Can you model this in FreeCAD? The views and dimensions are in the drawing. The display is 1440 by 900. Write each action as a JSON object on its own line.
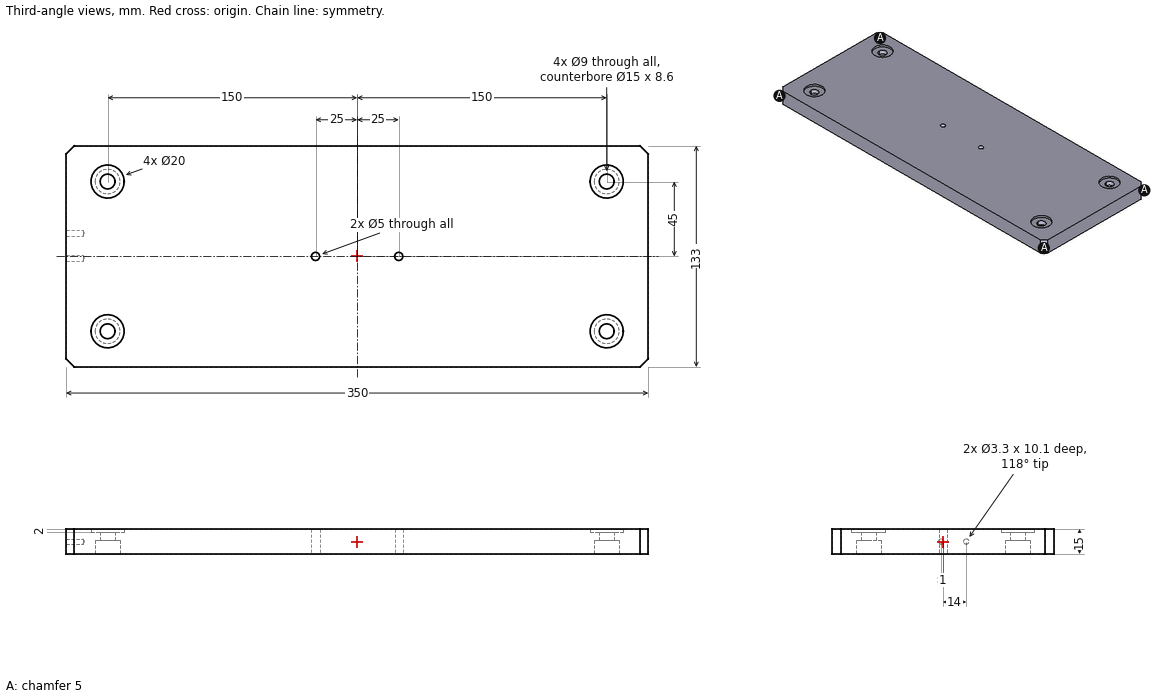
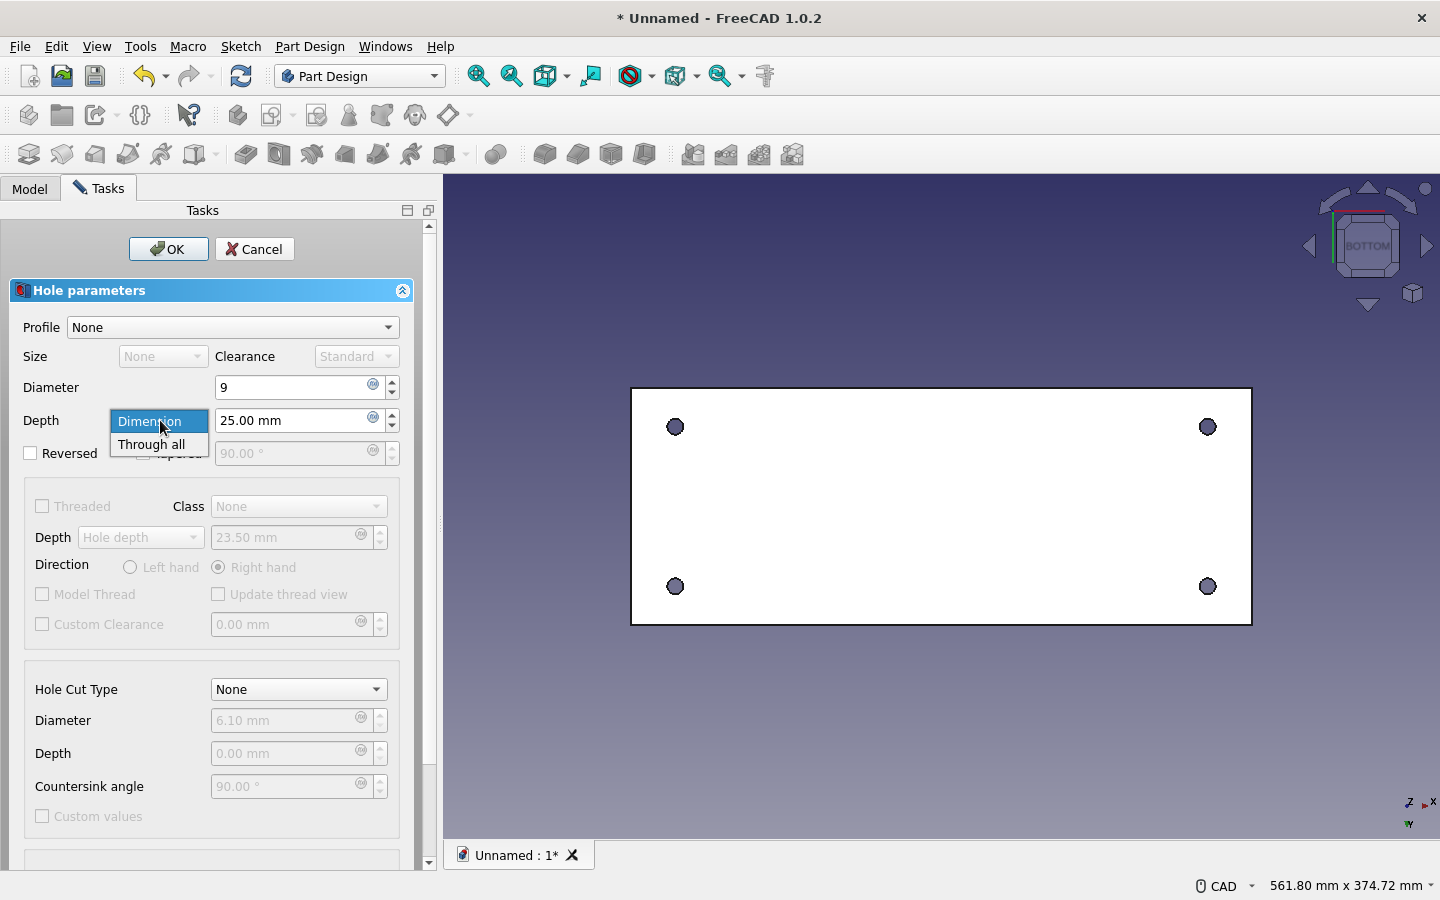
{"action": "left_click", "coordinate": [158, 444]}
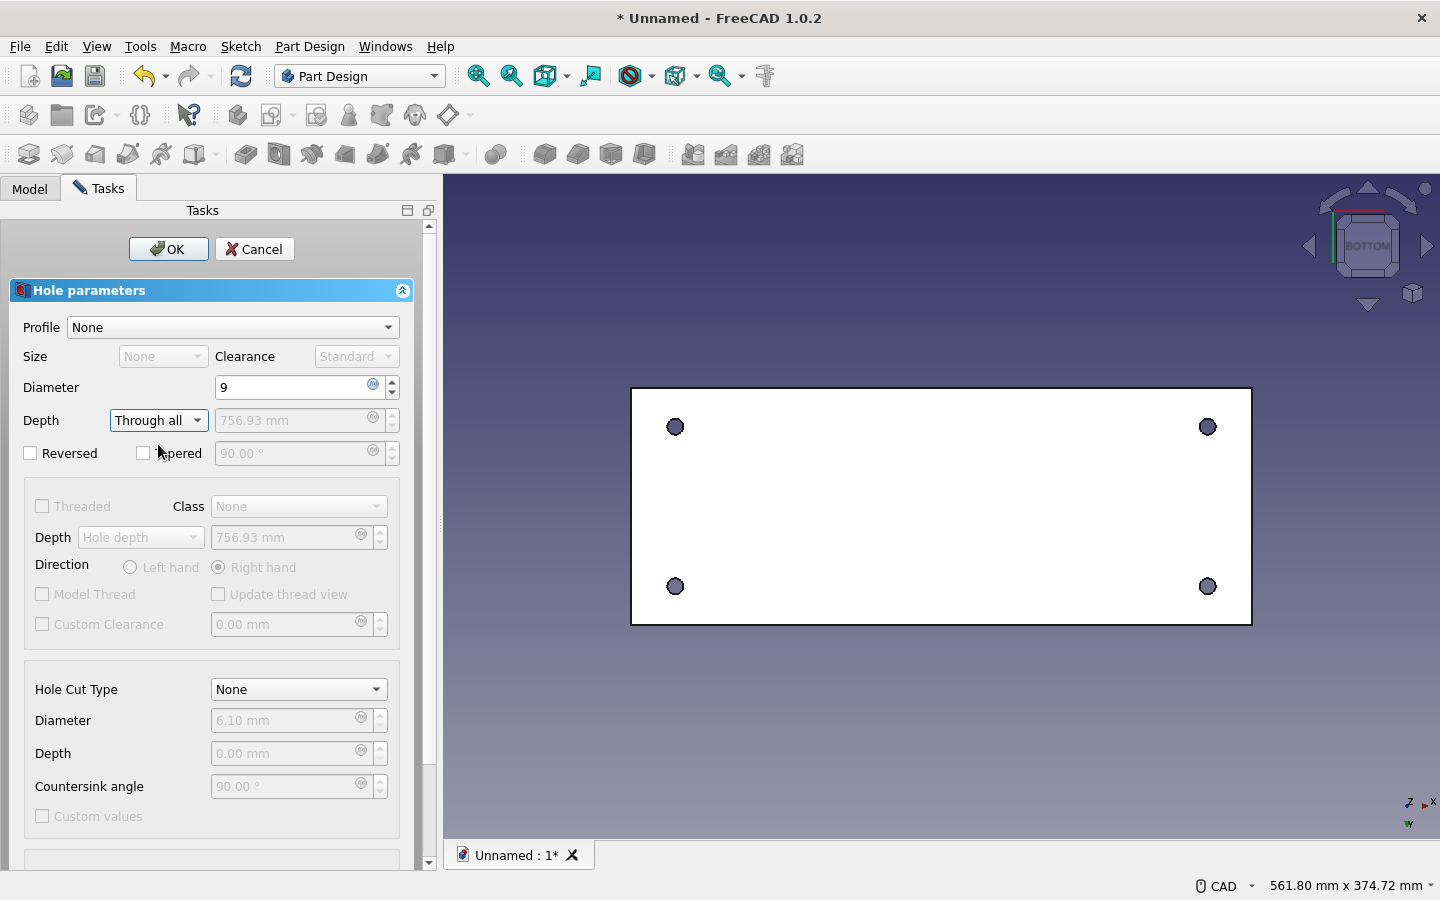
{"action": "left_click", "coordinate": [300, 690]}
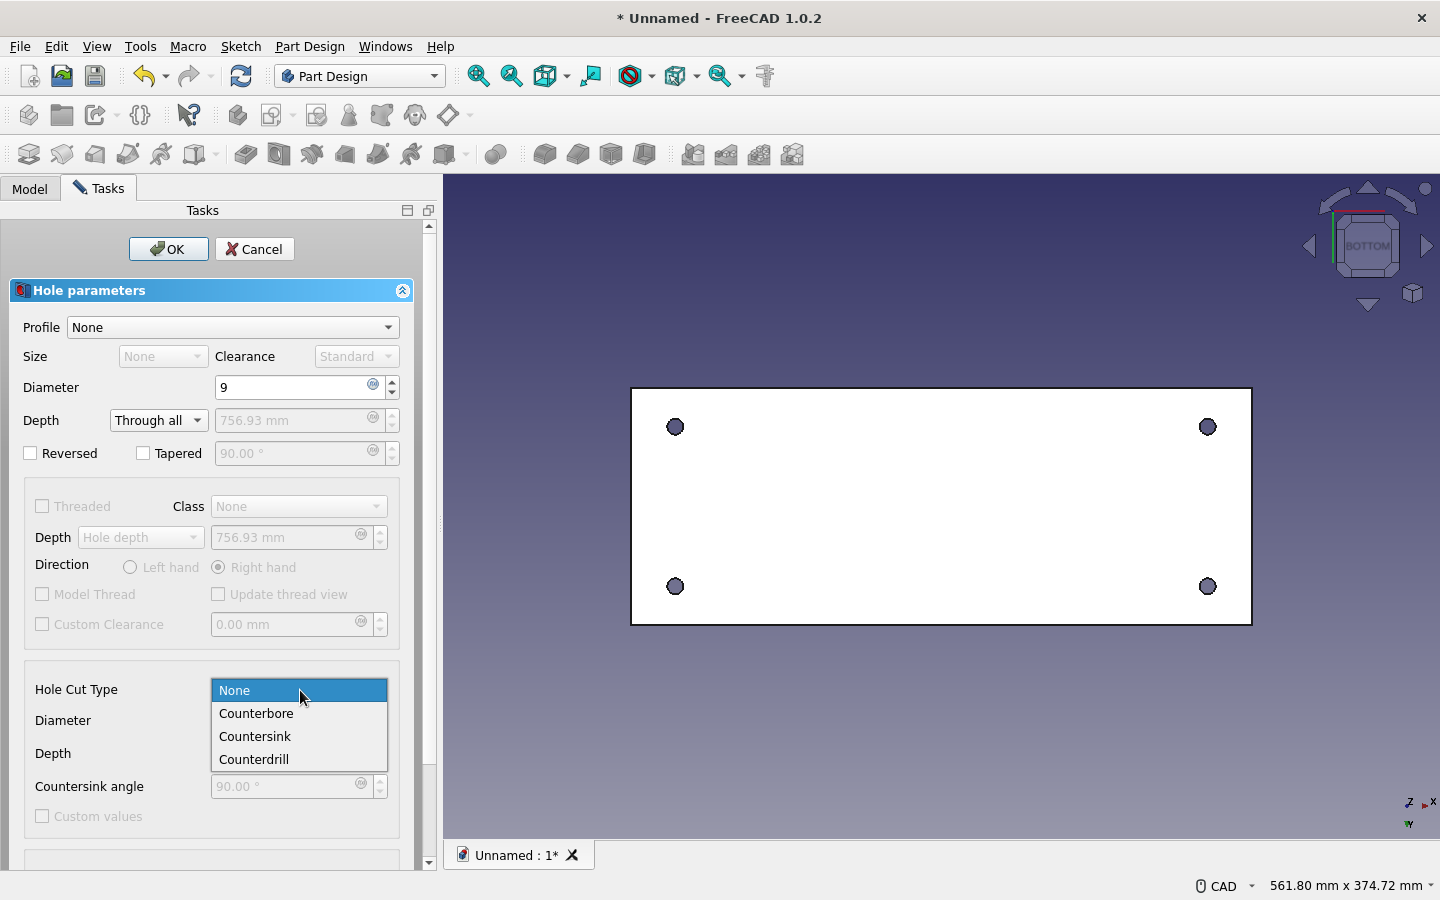
{"action": "left_click", "coordinate": [298, 714]}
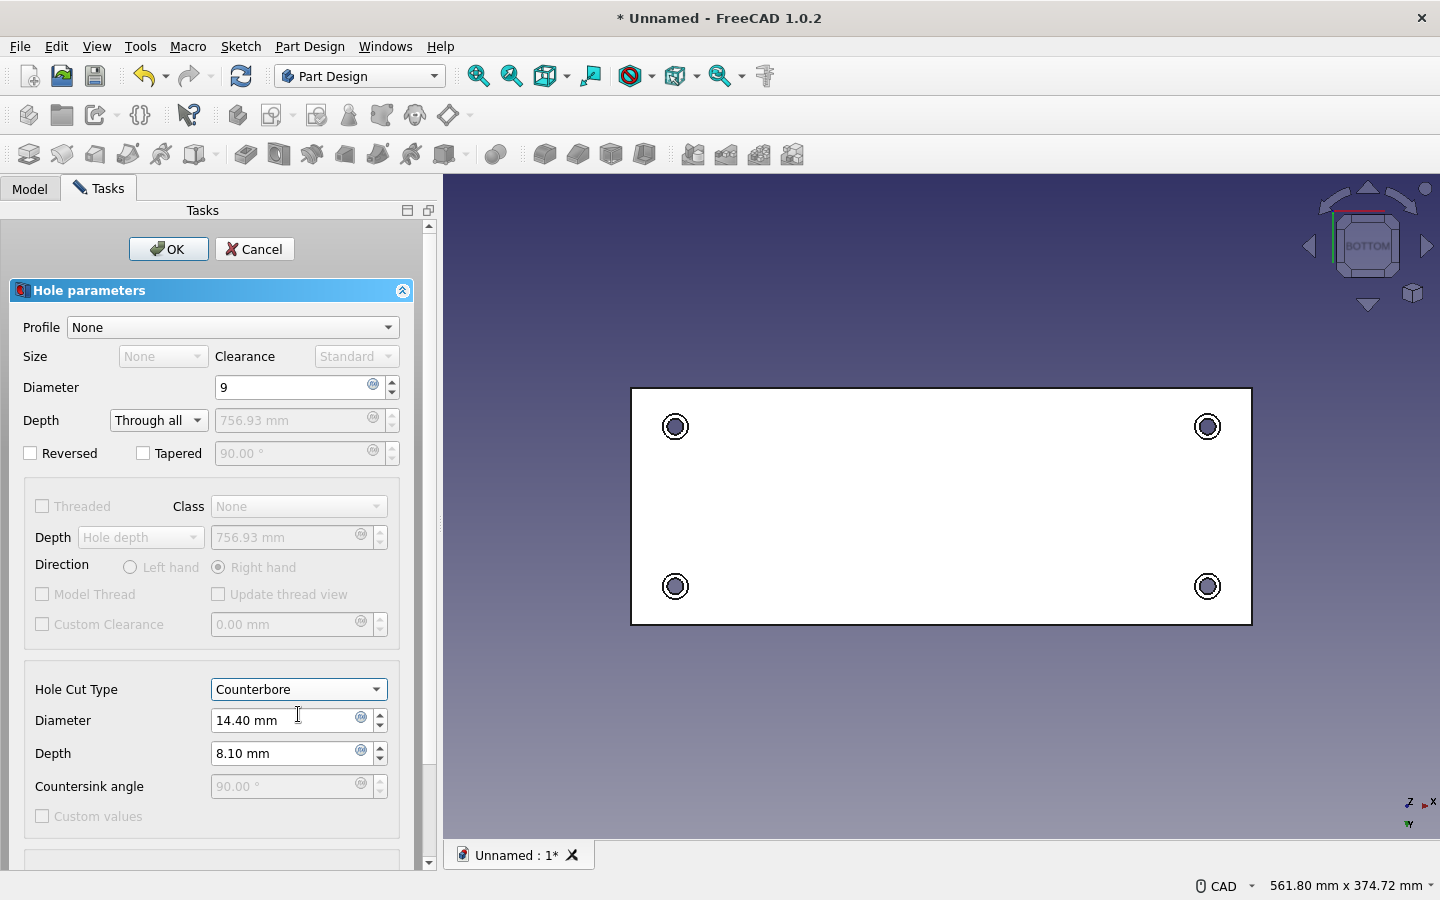
{"action": "triple_click", "coordinate": [292, 720]}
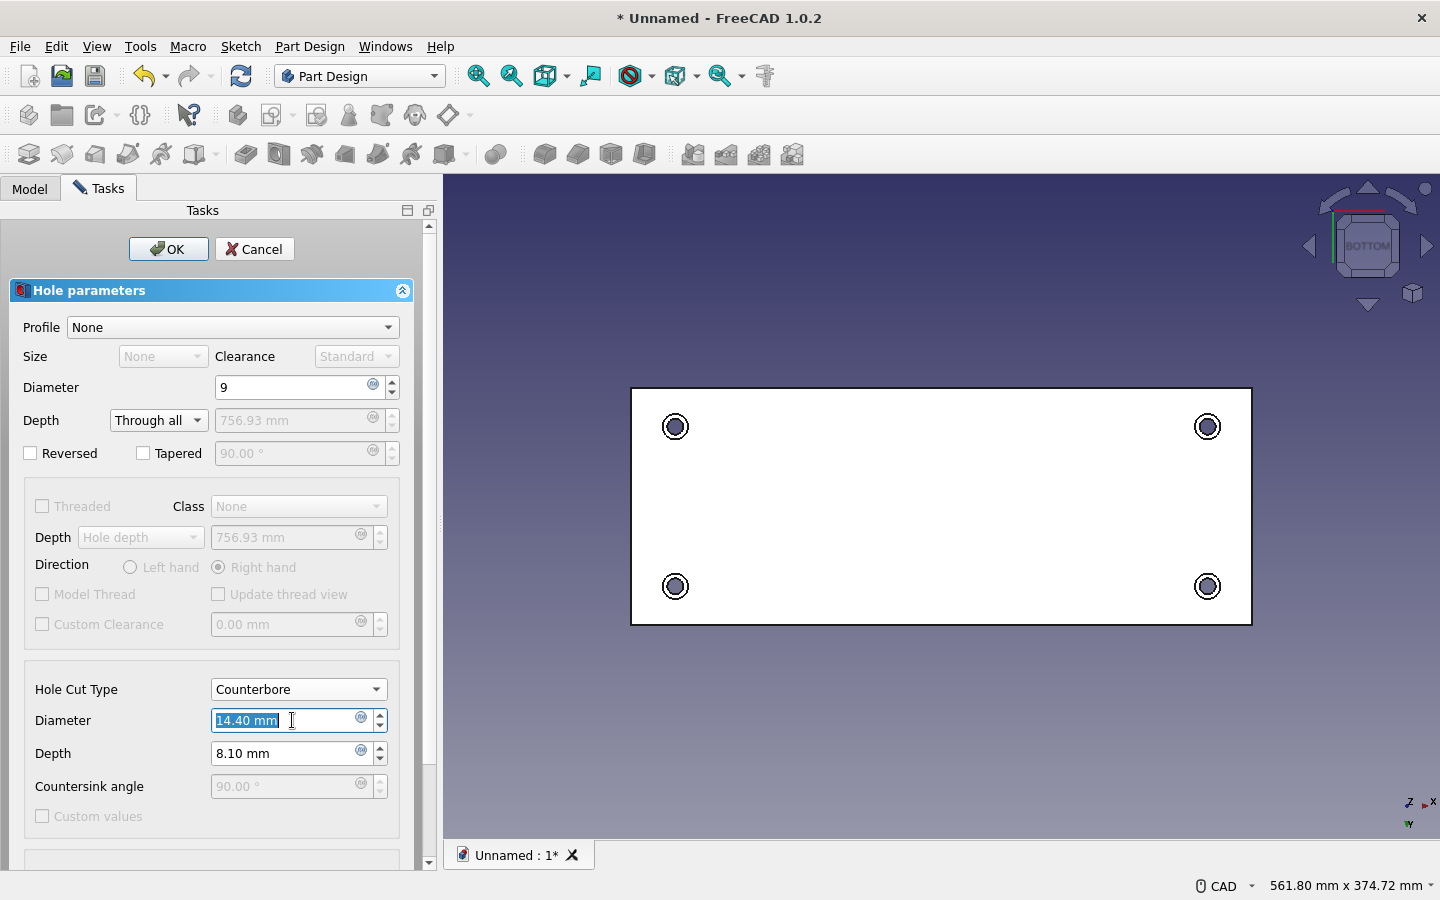
{"action": "type", "text": "15"}
{"action": "key", "text": "Tab"}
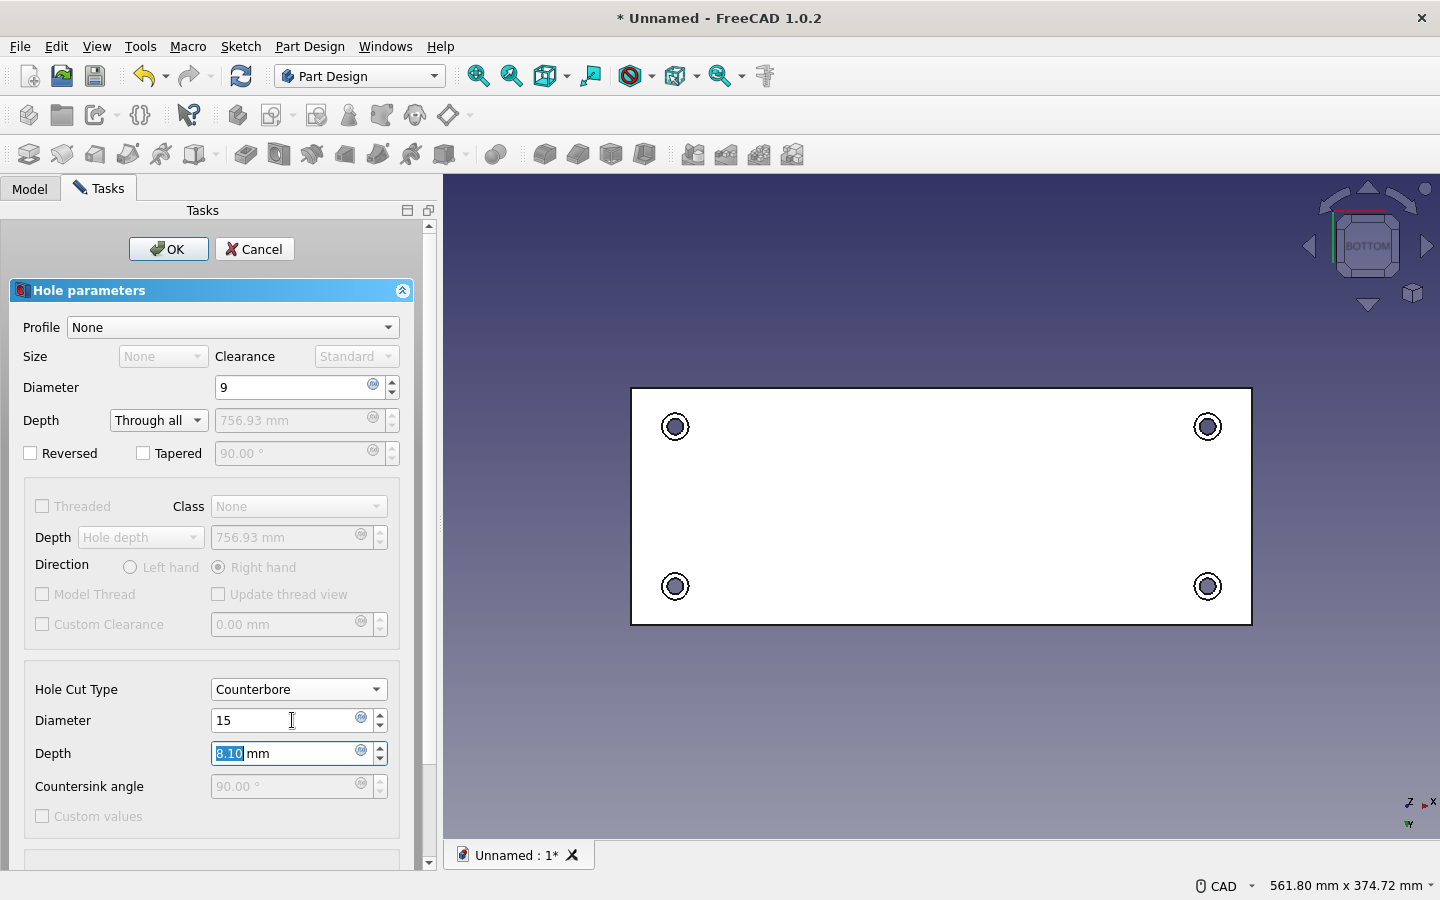
{"action": "type", "text": "8.6"}
{"action": "key", "text": "Tab"}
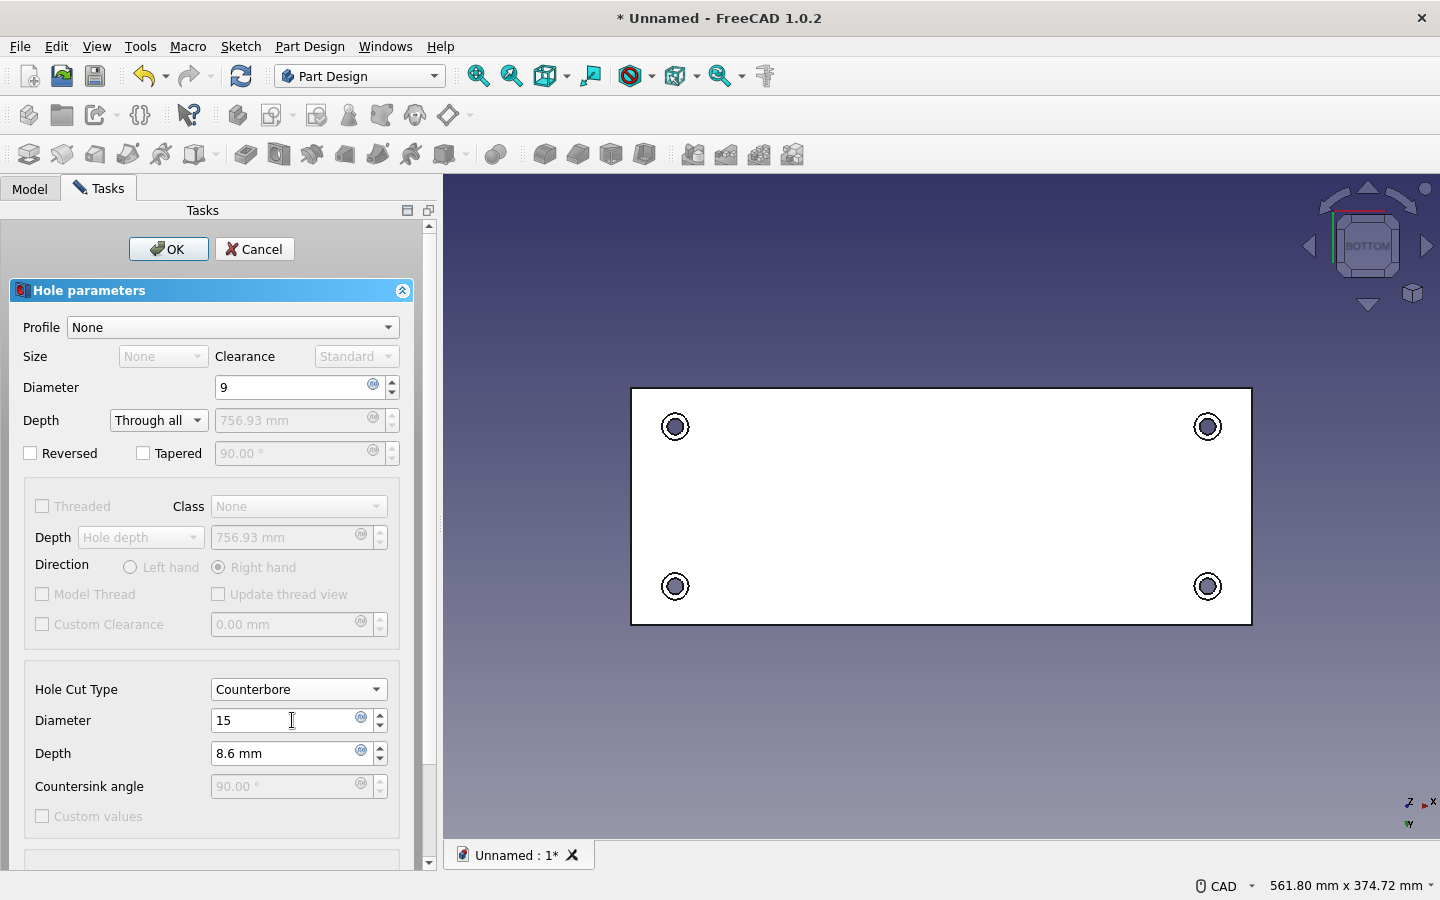
{"action": "left_click", "coordinate": [169, 249]}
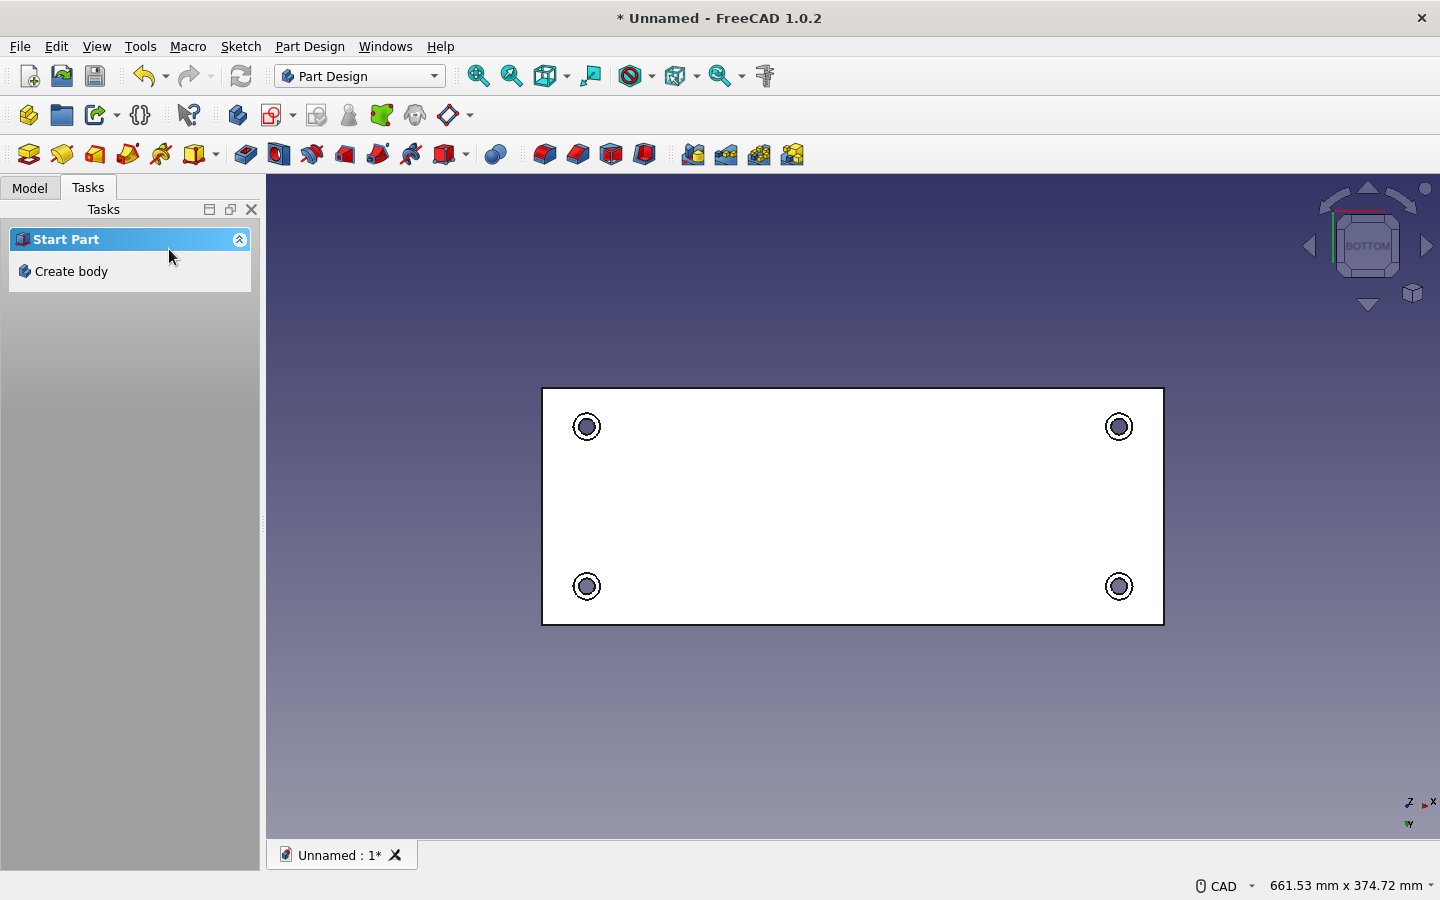
{"action": "key", "text": "0"}